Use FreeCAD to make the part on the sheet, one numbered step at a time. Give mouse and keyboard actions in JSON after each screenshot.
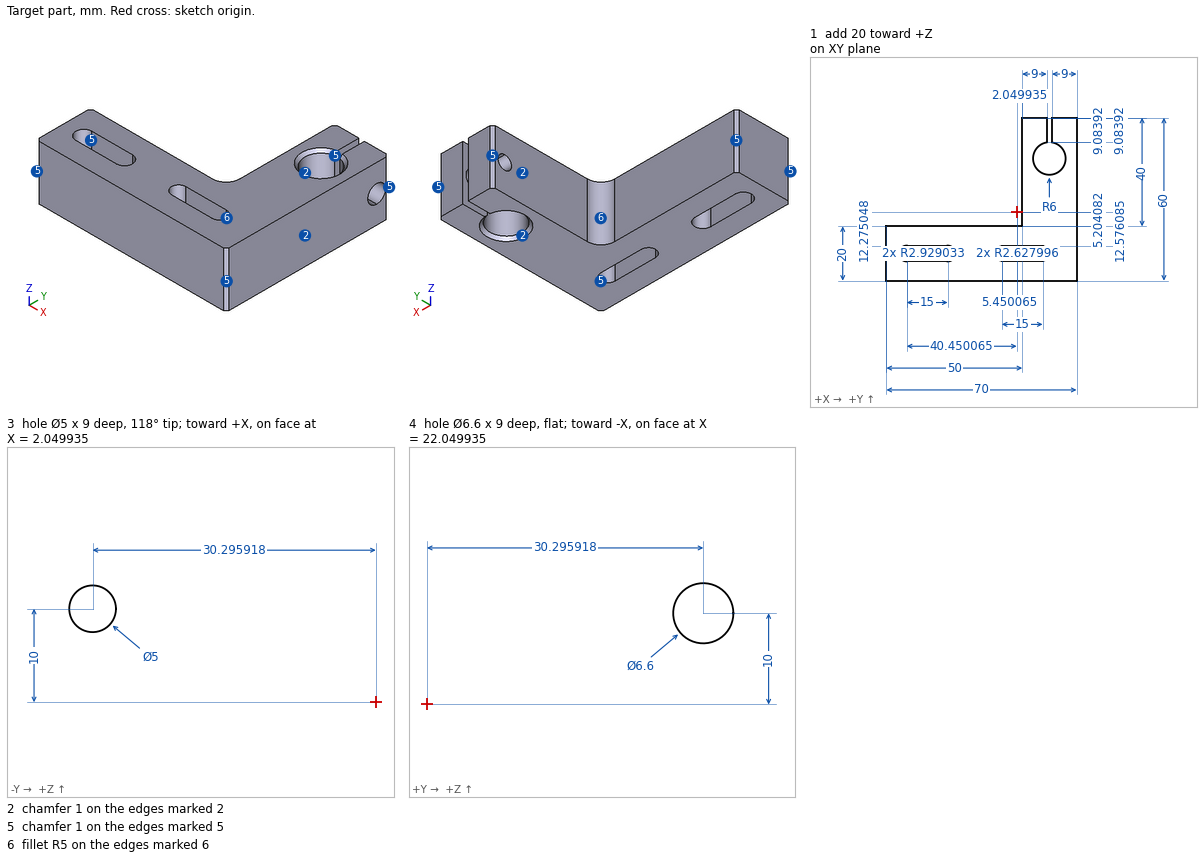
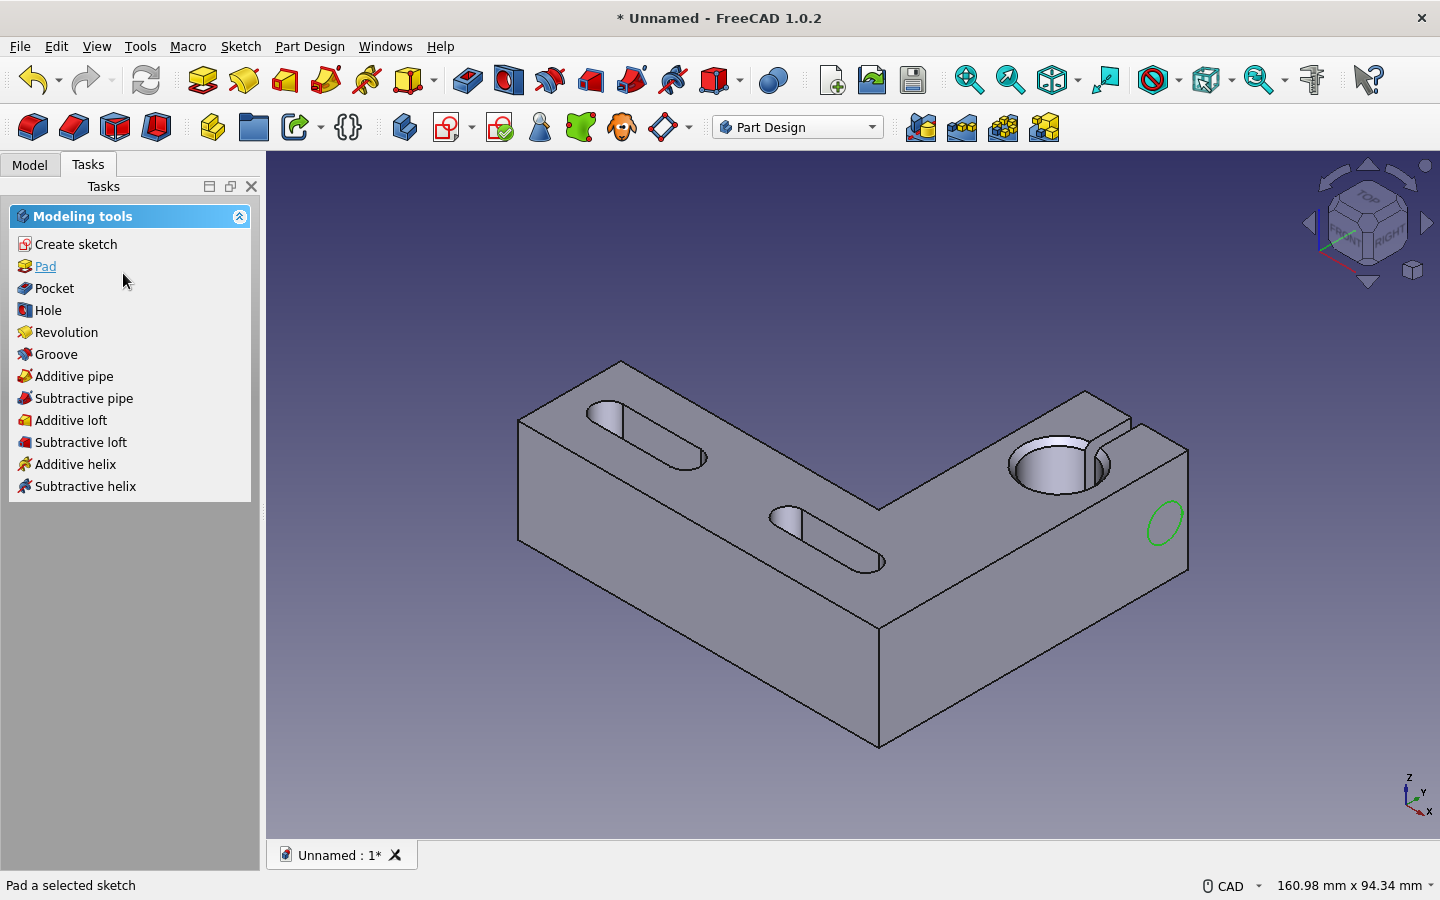
{"action": "left_click", "coordinate": [509, 80]}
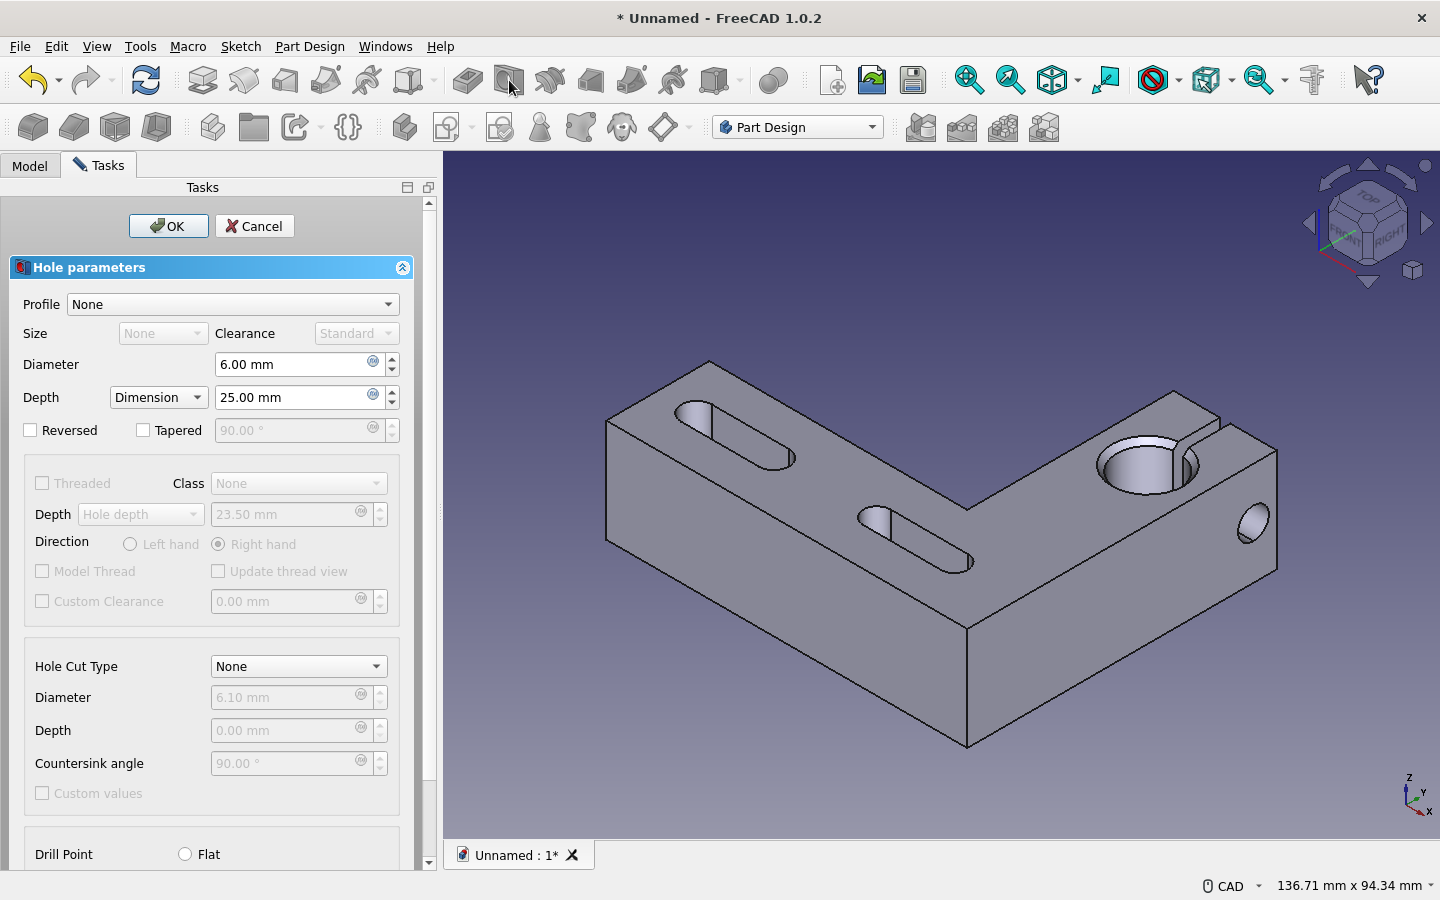
{"action": "triple_click", "coordinate": [300, 364]}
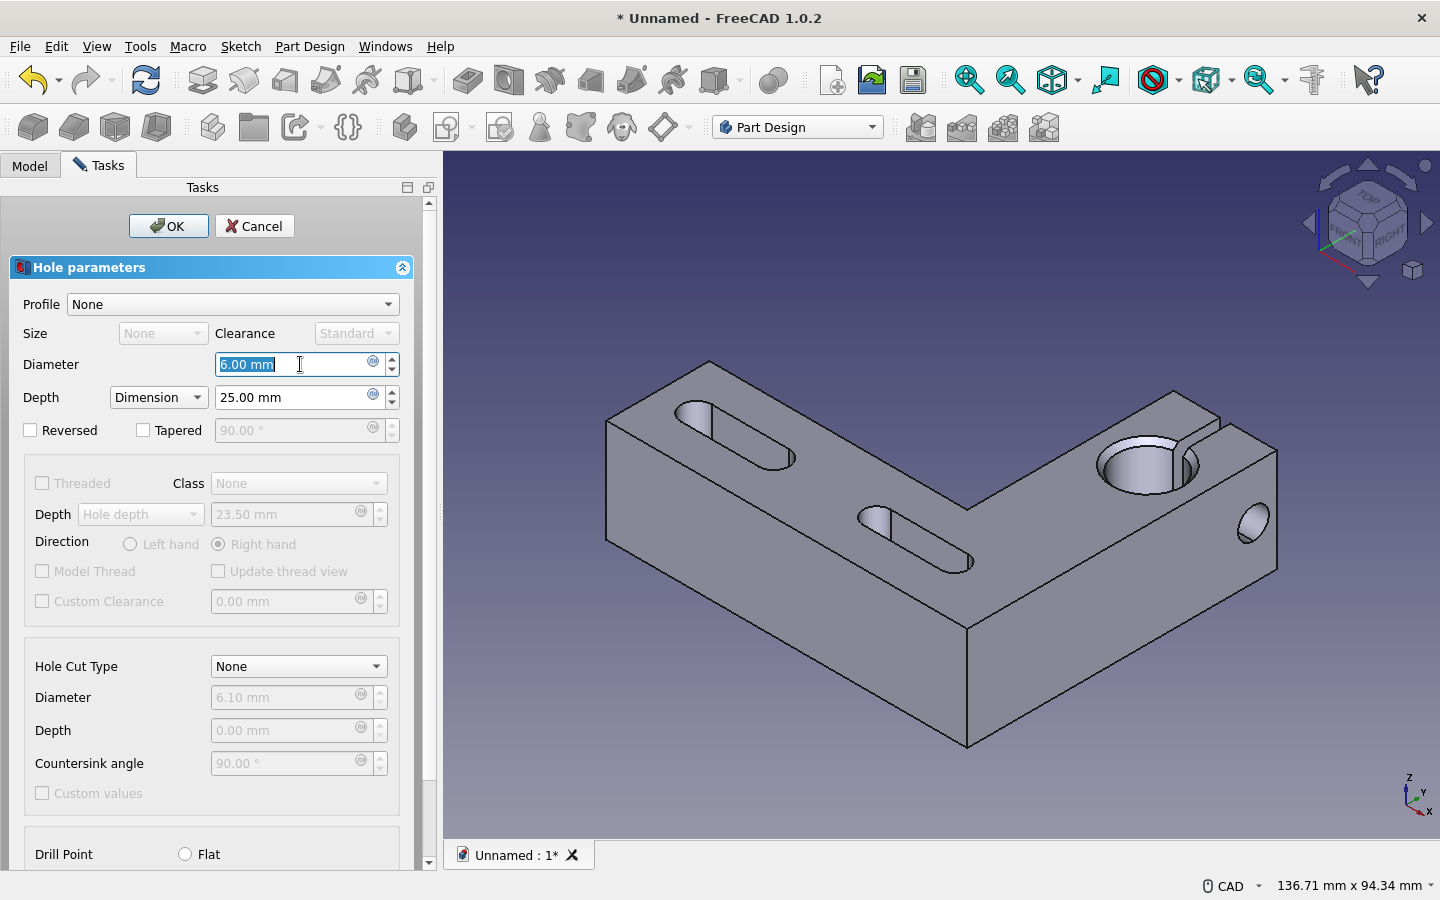
{"action": "type", "text": "6.6"}
{"action": "key", "text": "Tab"}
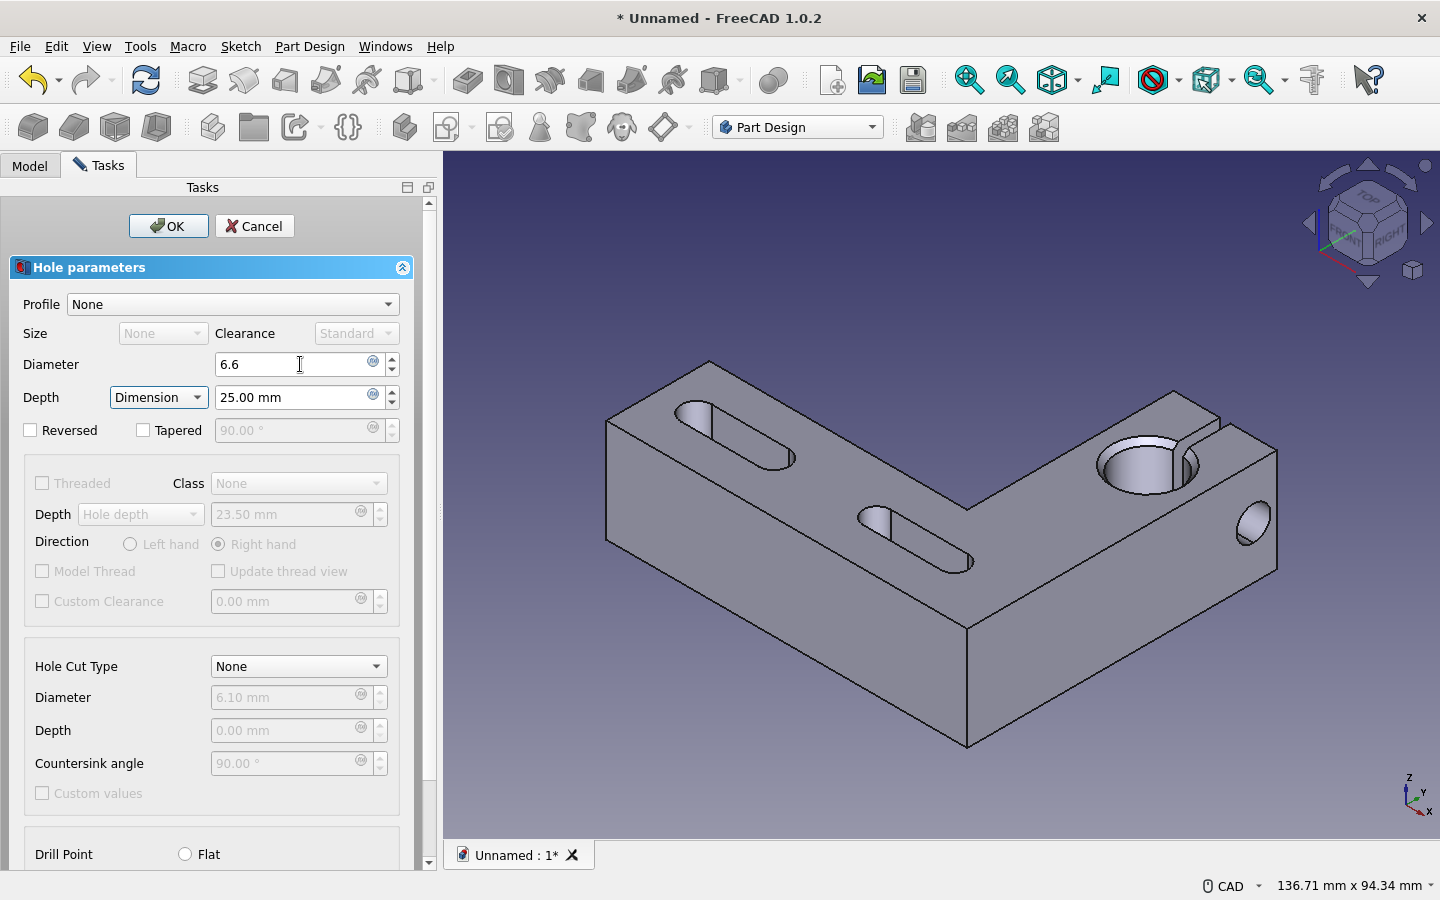
{"action": "triple_click", "coordinate": [300, 398]}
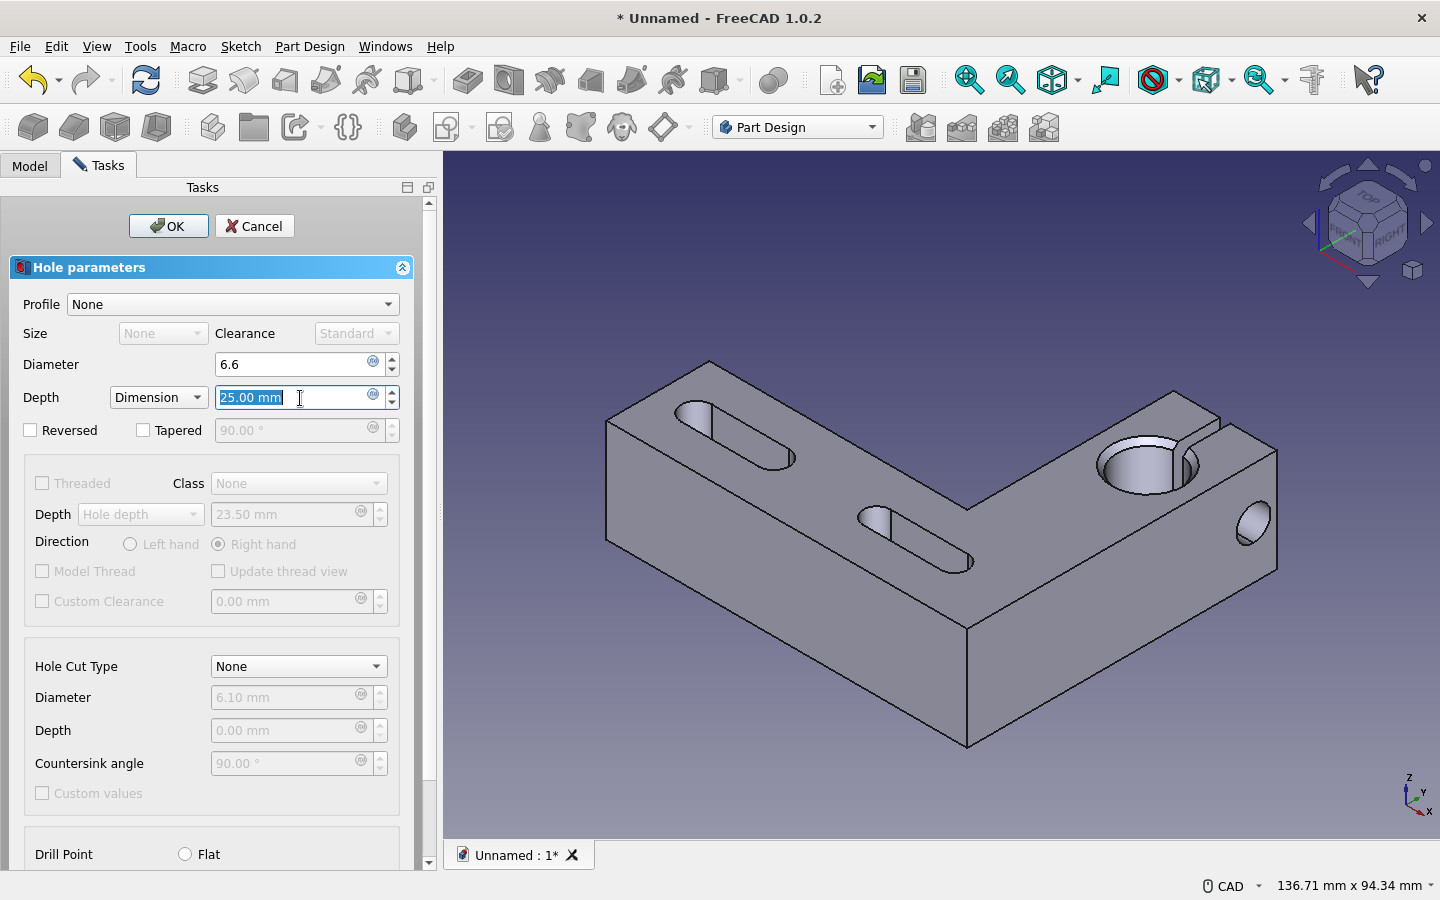
{"action": "type", "text": "9"}
{"action": "key", "text": "Tab"}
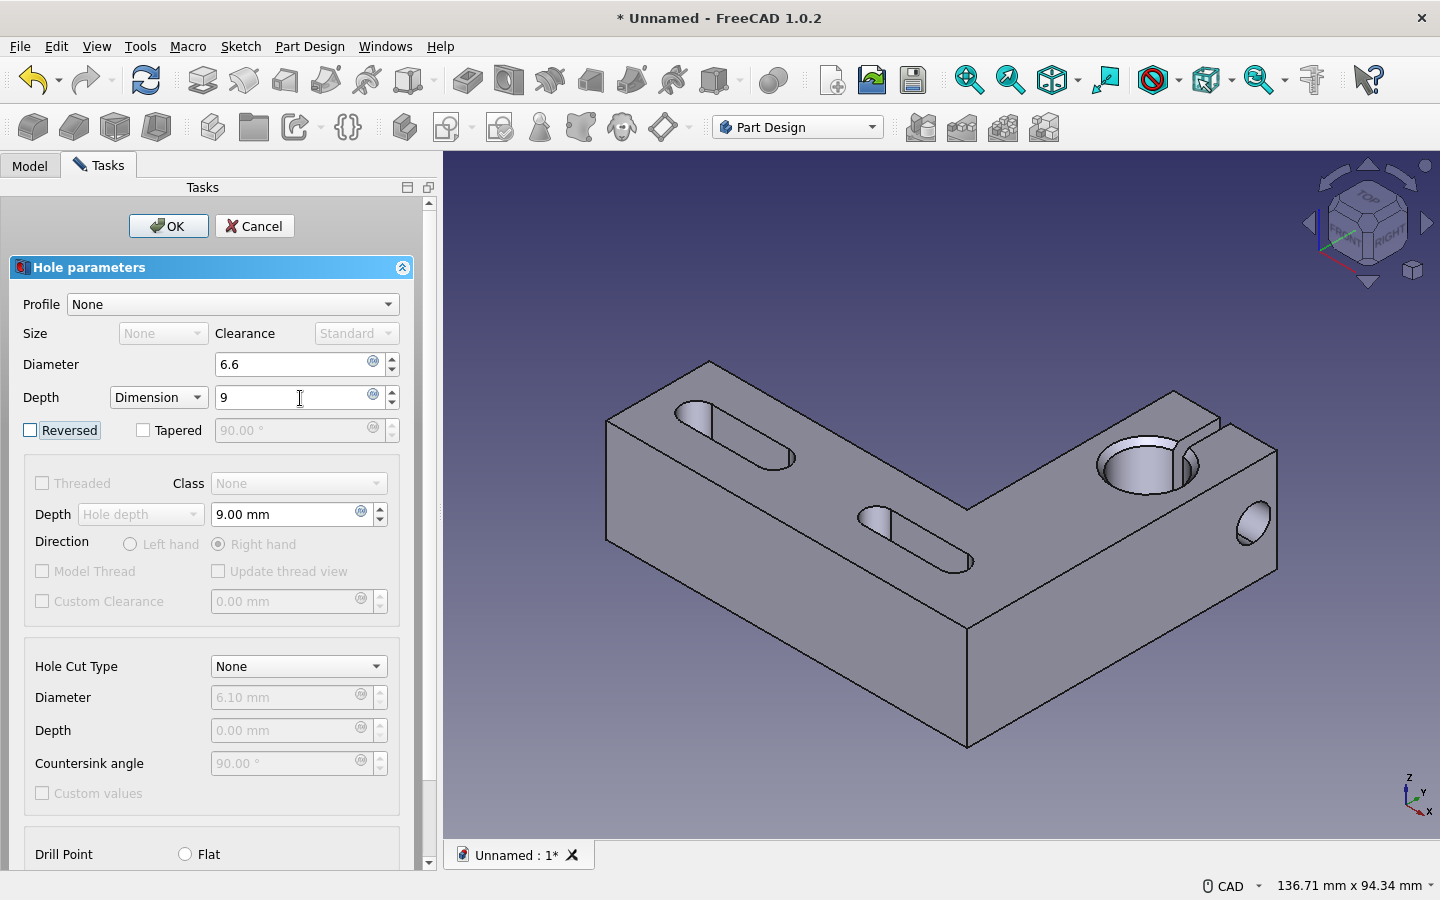
{"action": "left_click", "coordinate": [186, 852]}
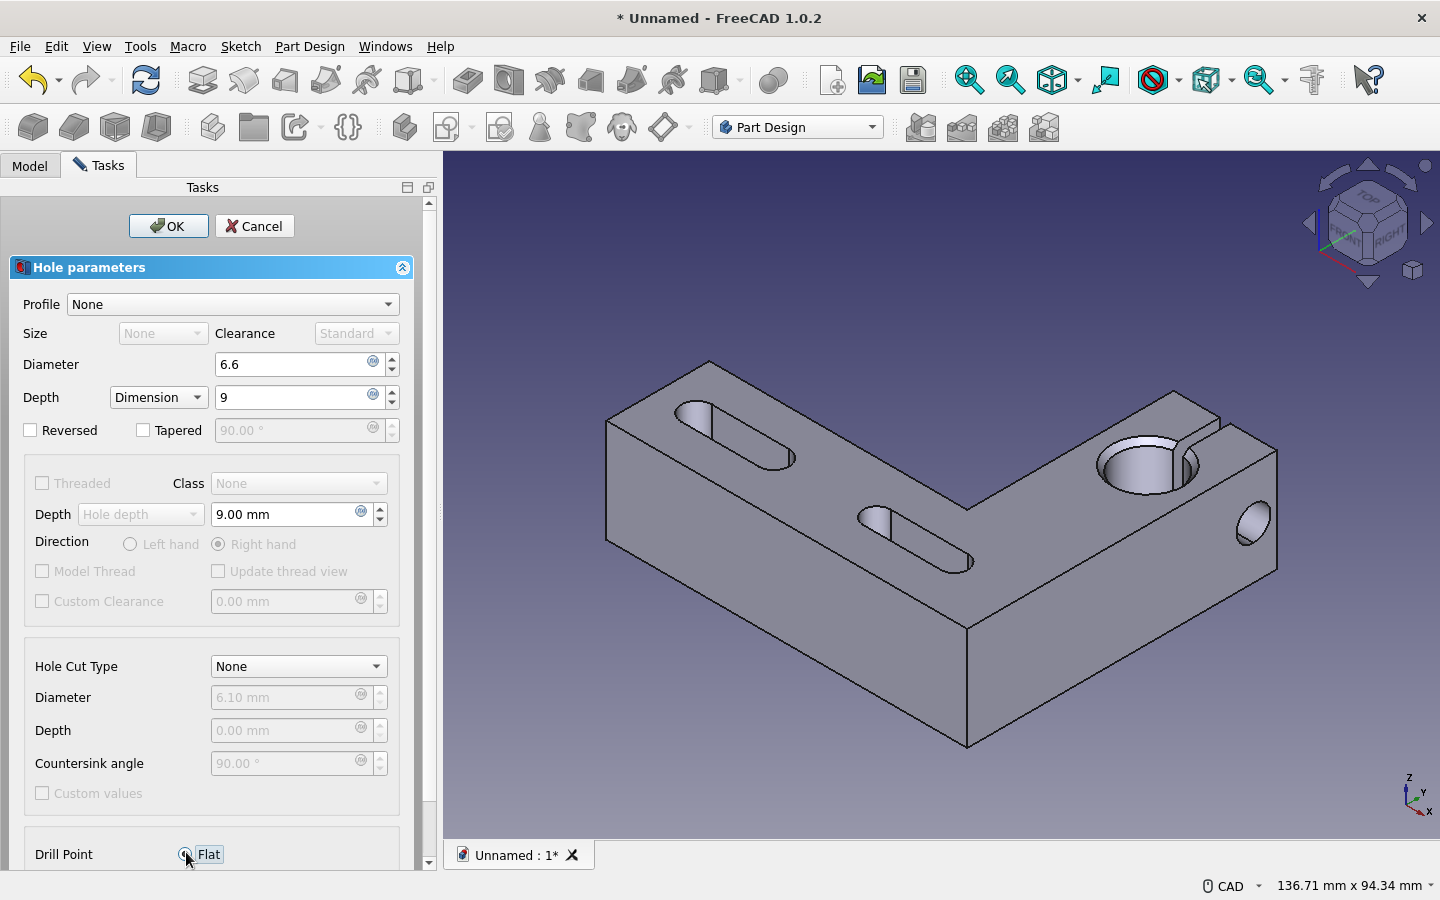
{"action": "left_click", "coordinate": [169, 226]}